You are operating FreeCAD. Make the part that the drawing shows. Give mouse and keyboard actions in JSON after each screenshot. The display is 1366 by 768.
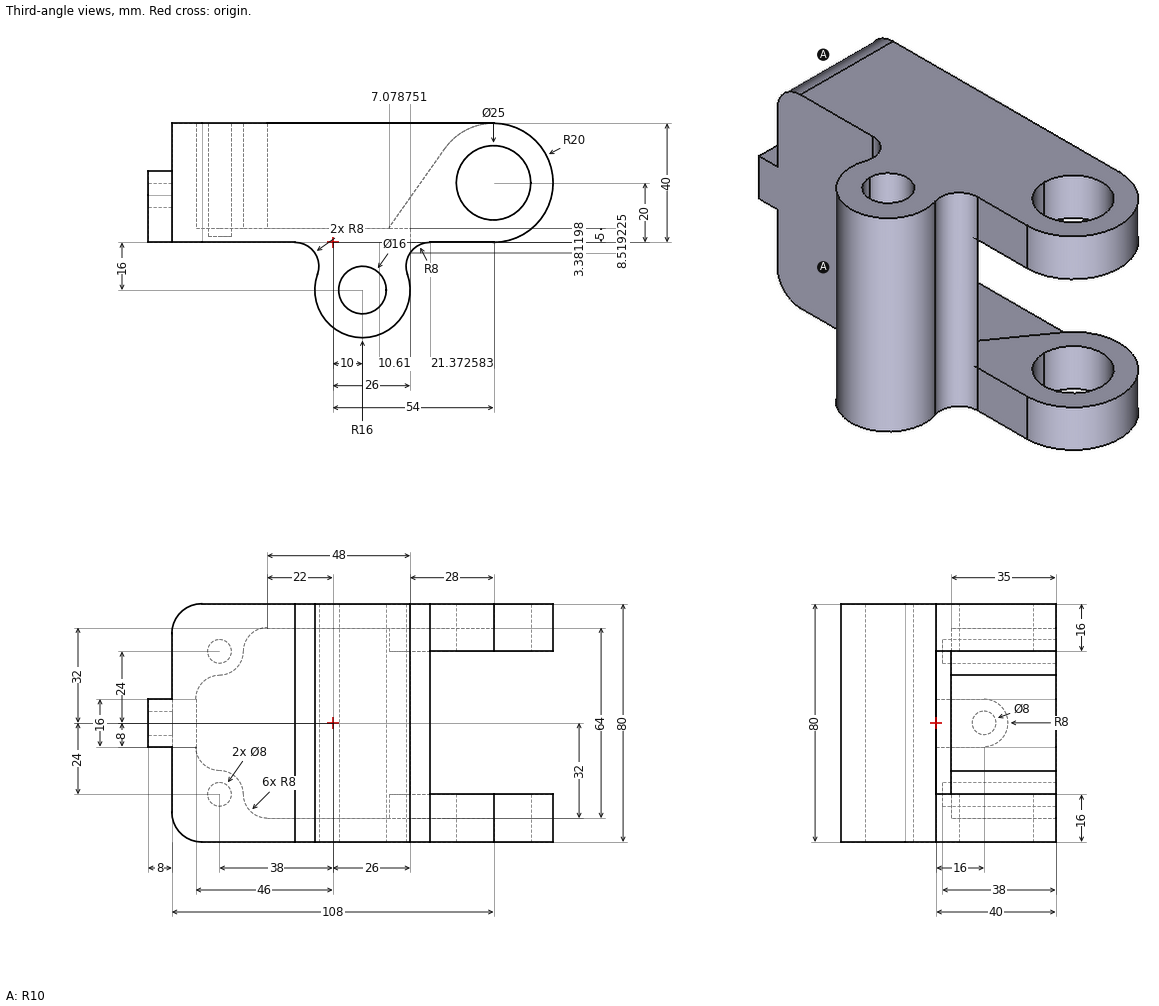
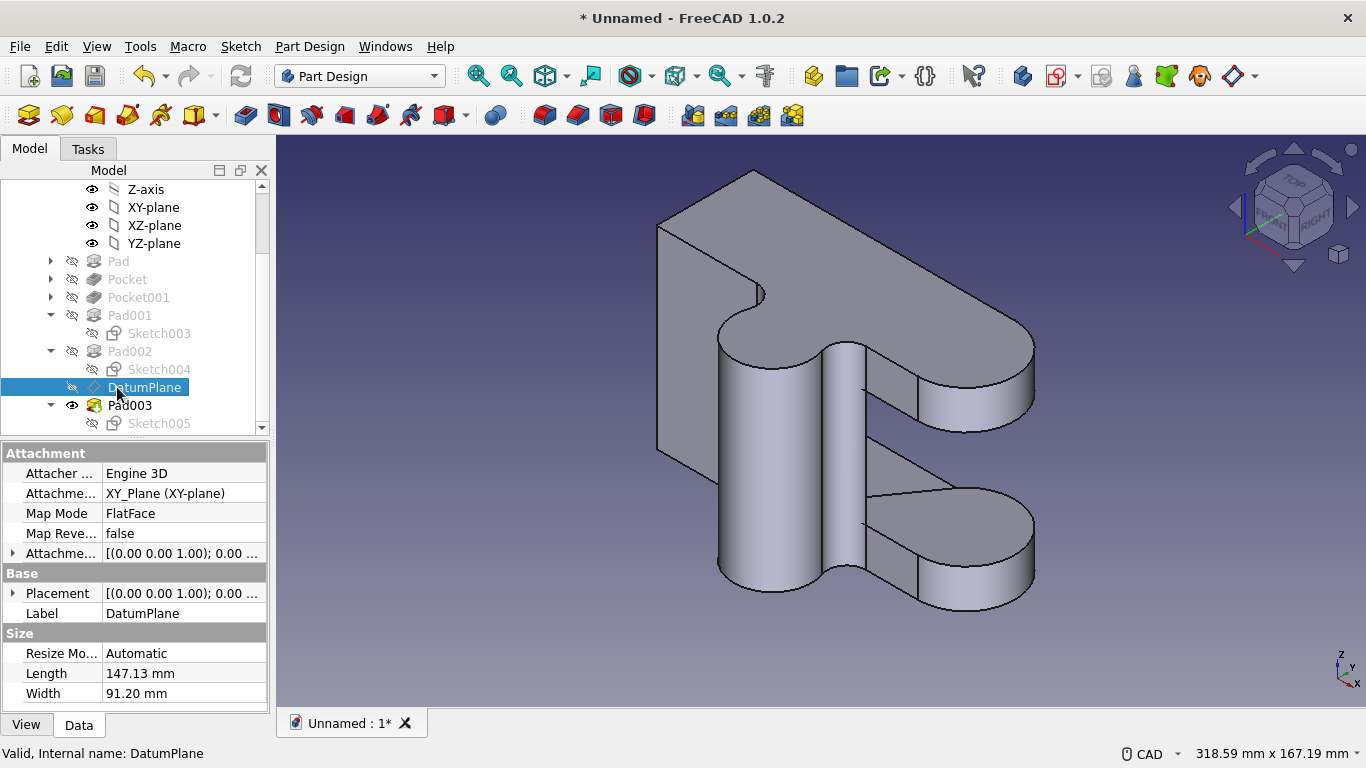
{"action": "left_click", "coordinate": [846, 294]}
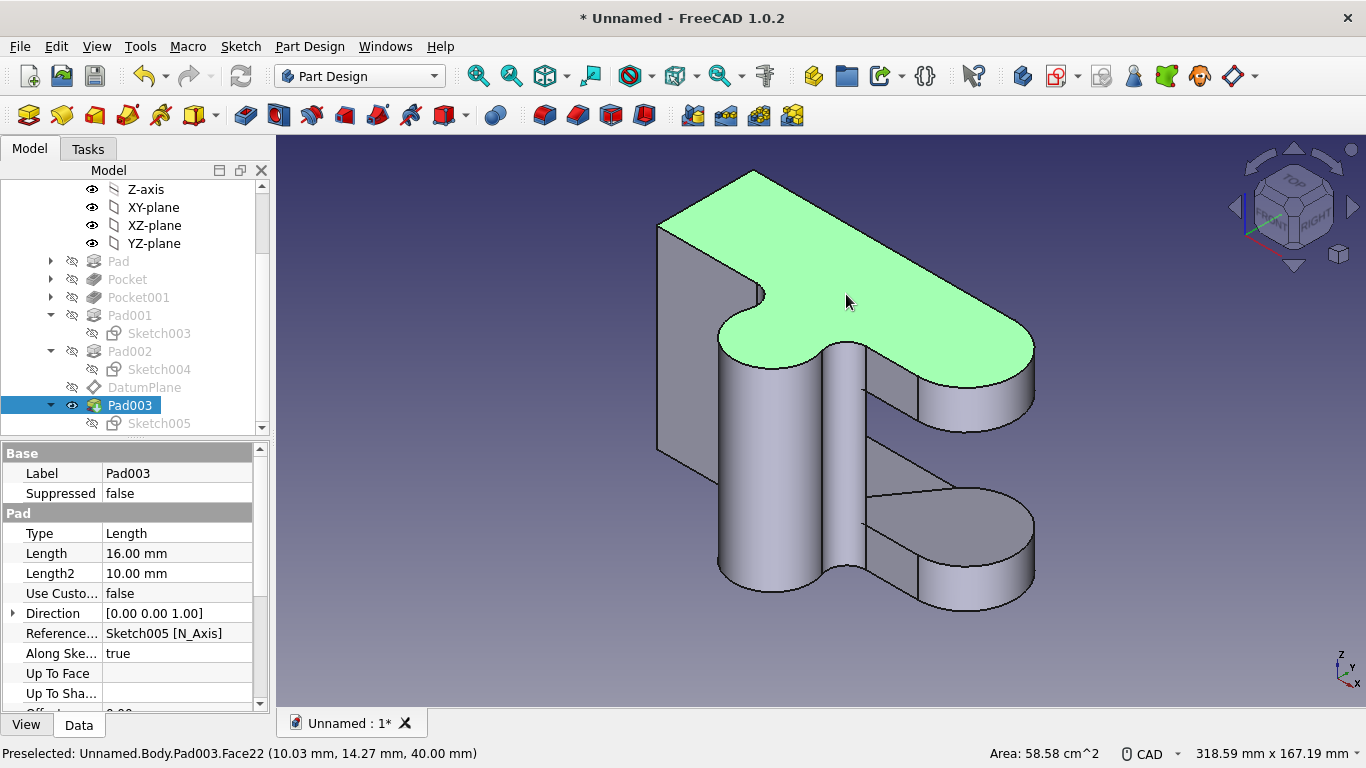
{"action": "left_click", "coordinate": [1056, 76]}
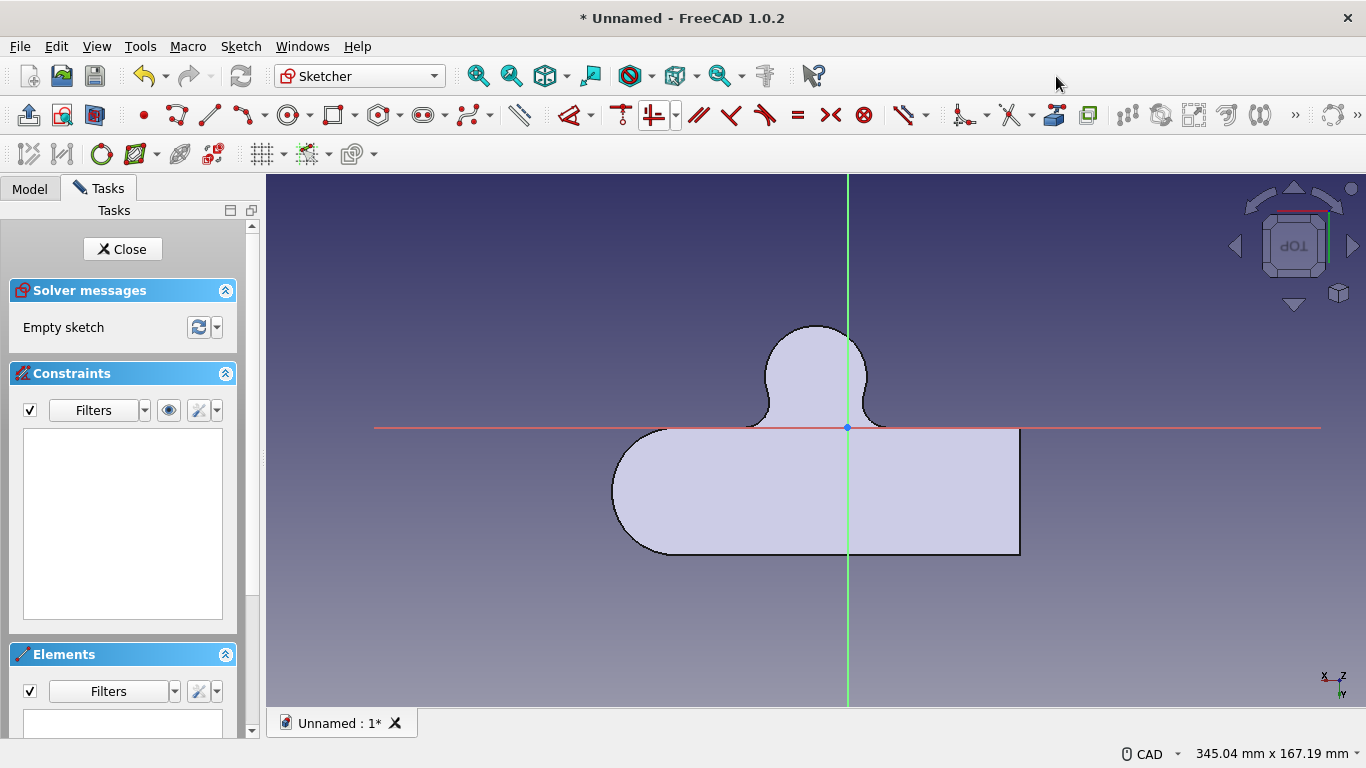
{"action": "scroll", "coordinate": [735, 442], "scroll_direction": "up", "scroll_amount": 3}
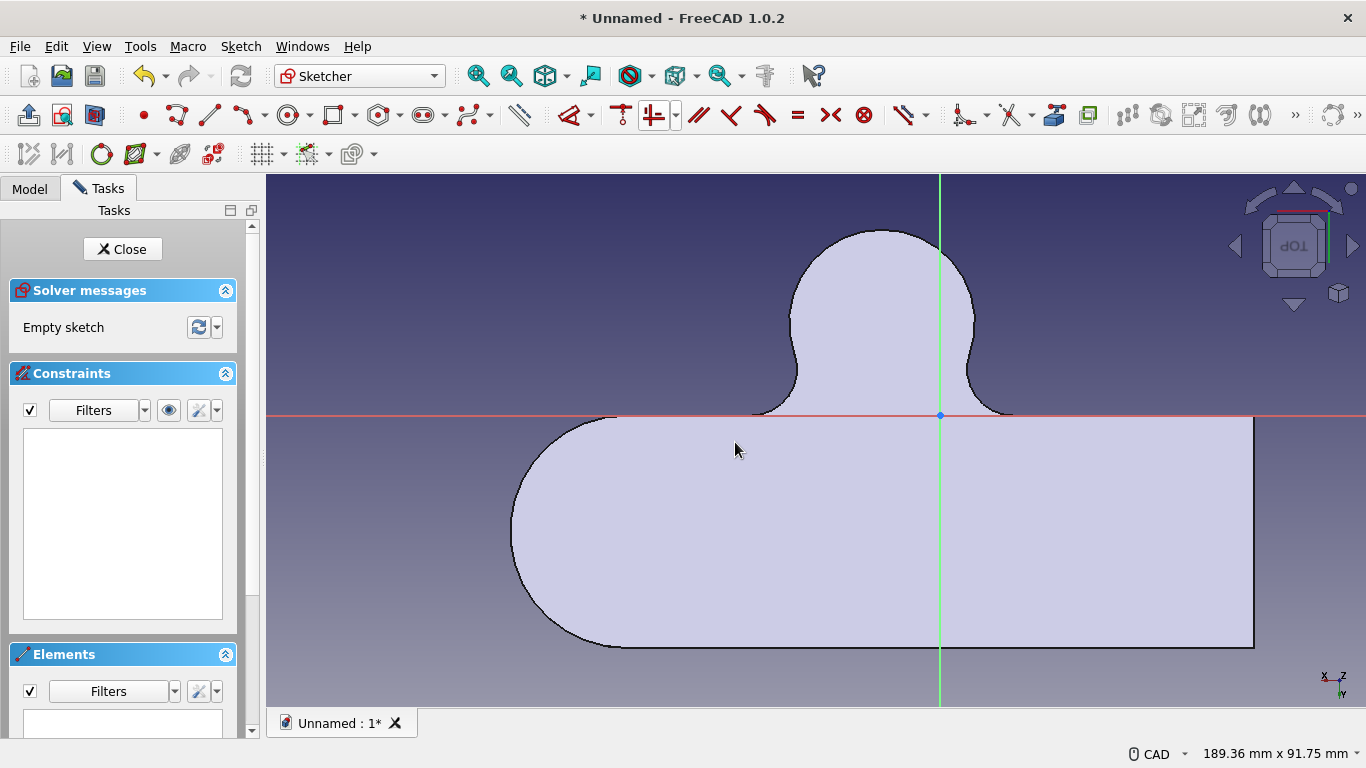
{"action": "key", "text": "g c"}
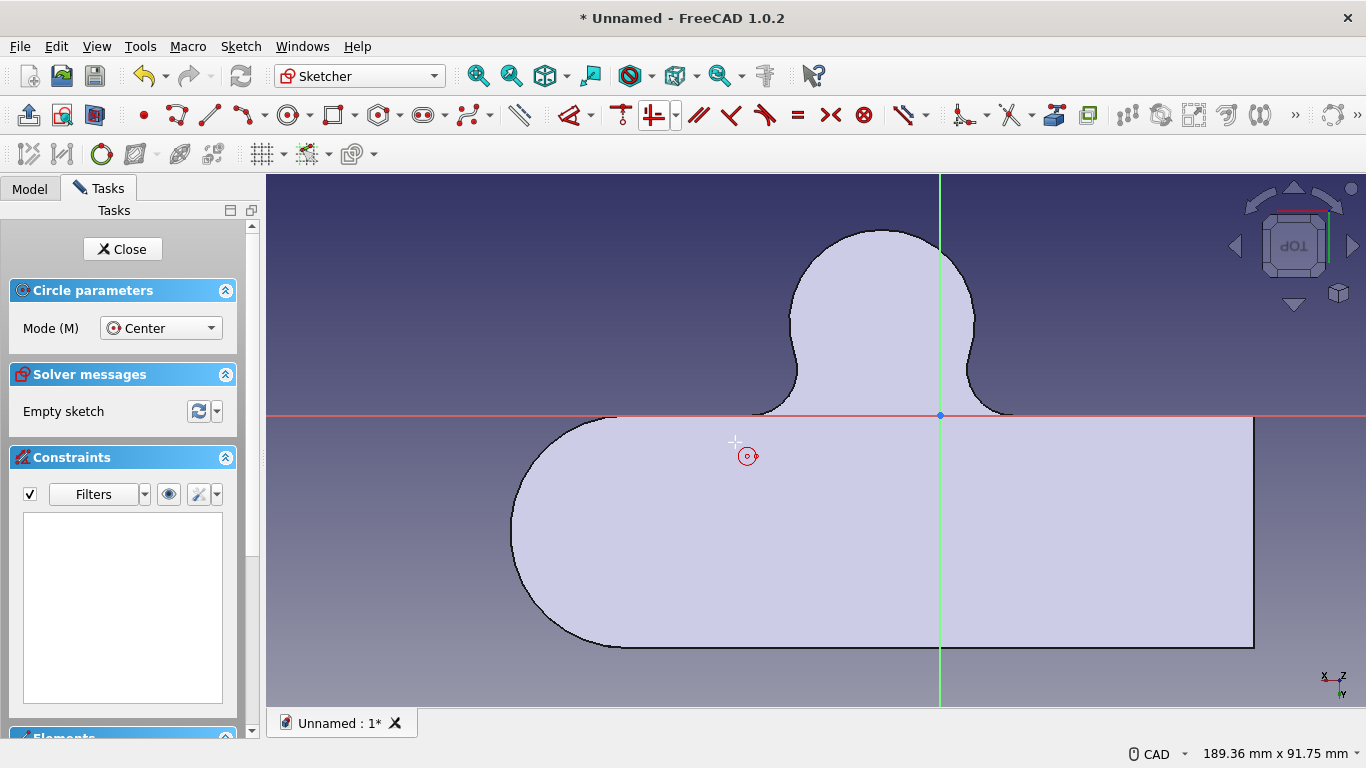
{"action": "left_click", "coordinate": [626, 532]}
{"action": "mouse_move", "coordinate": [678, 480]}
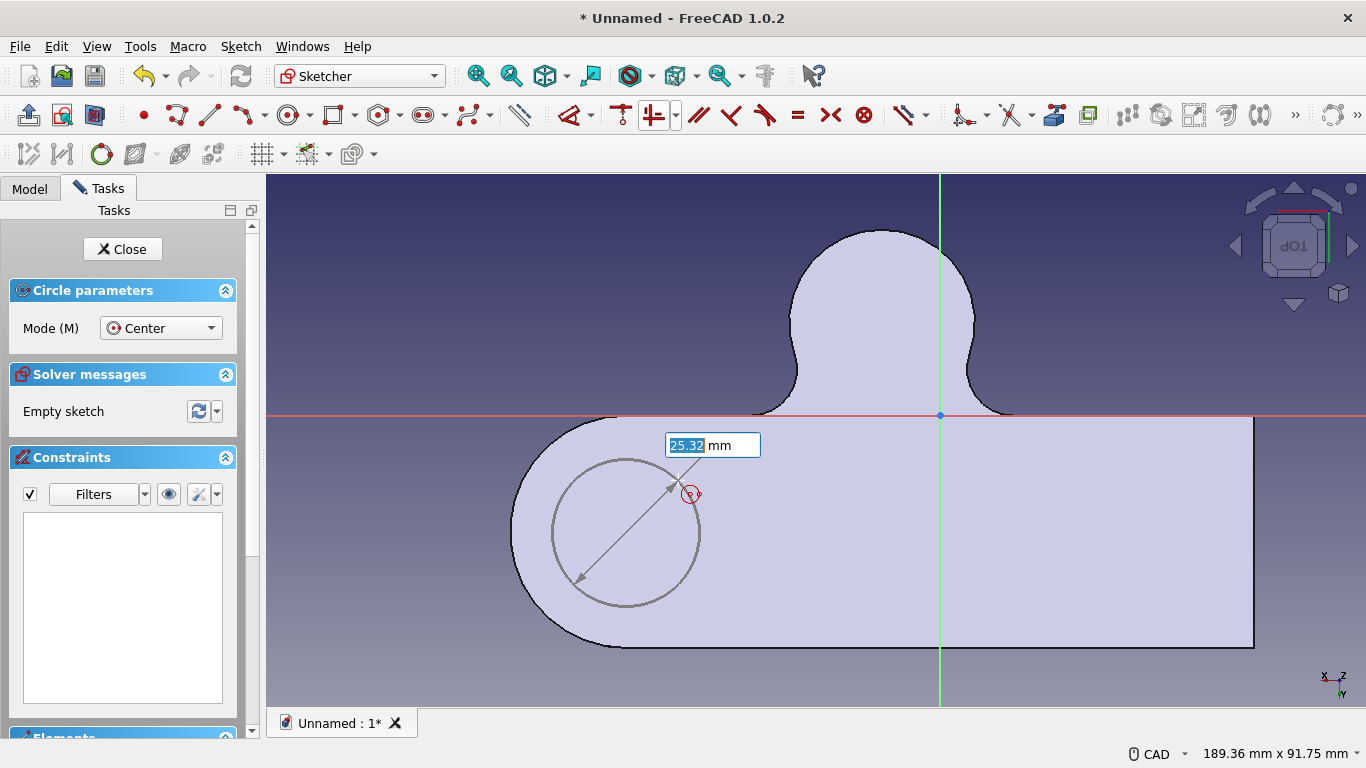
{"action": "type", "text": "25"}
{"action": "key", "text": "Return"}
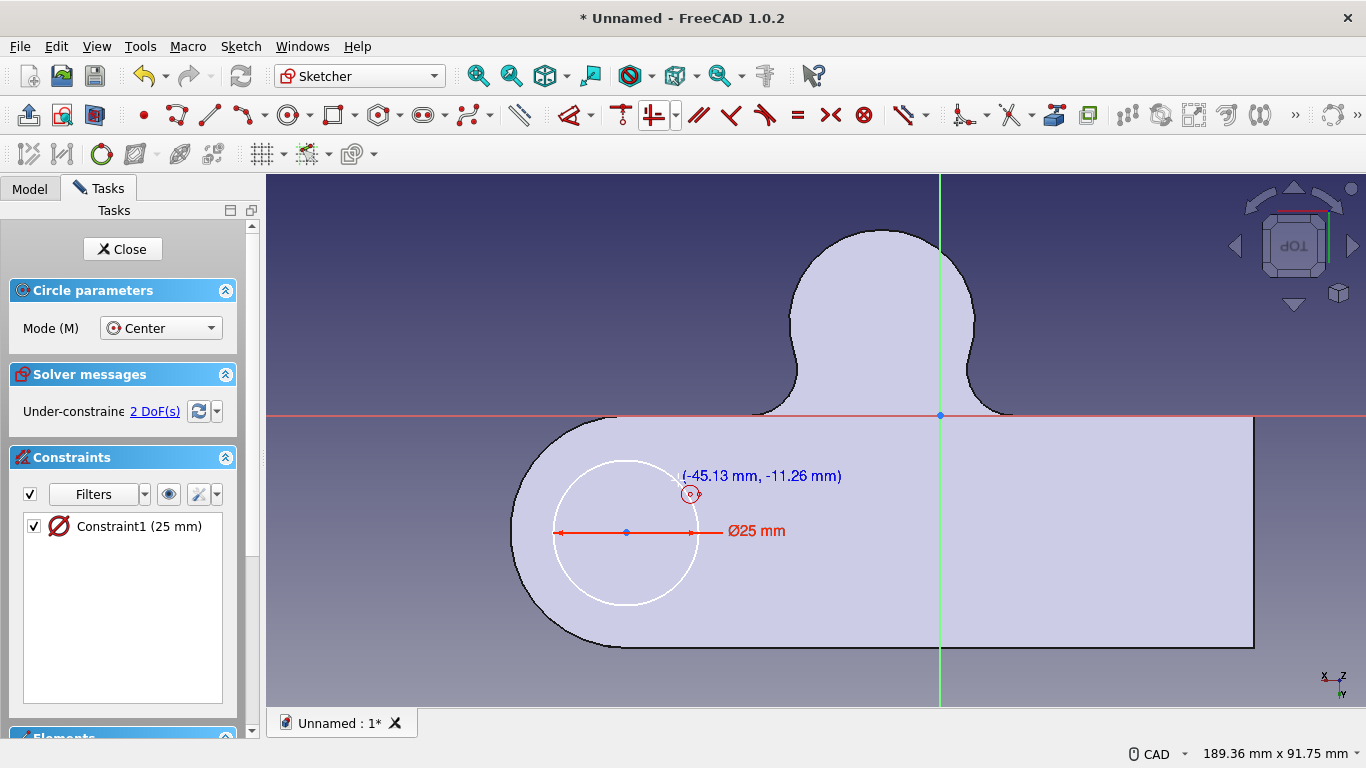
{"action": "left_click", "coordinate": [882, 323]}
{"action": "mouse_move", "coordinate": [915, 290]}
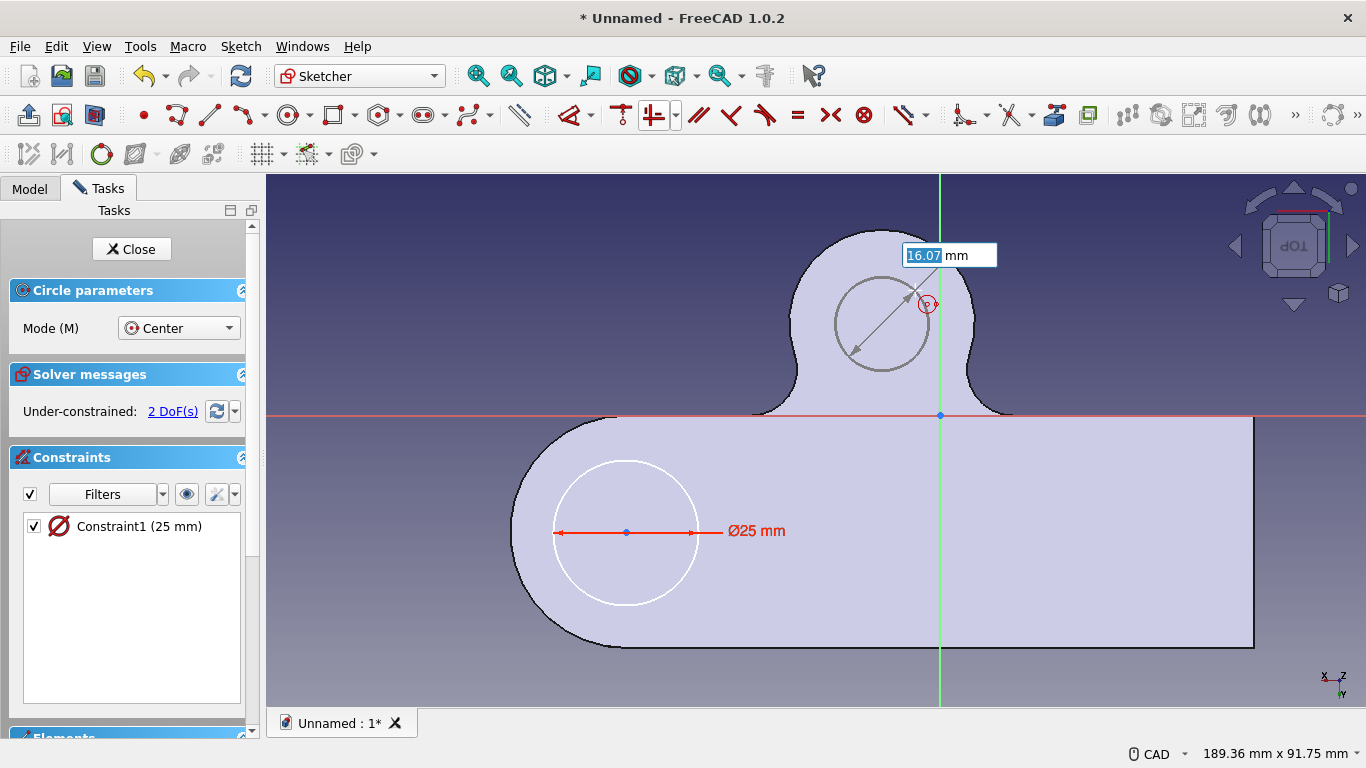
{"action": "type", "text": "16"}
{"action": "key", "text": "Return"}
{"action": "key", "text": "Escape"}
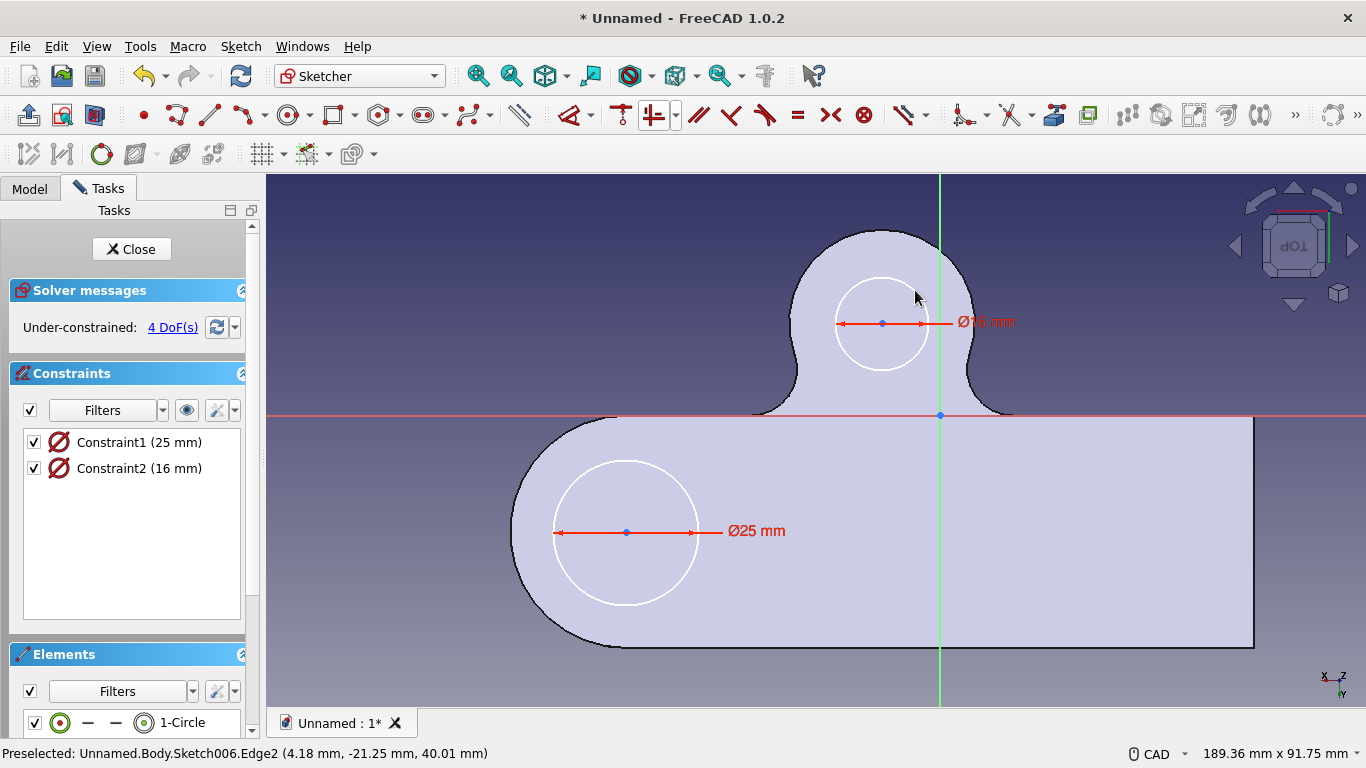
{"action": "left_click", "coordinate": [568, 116]}